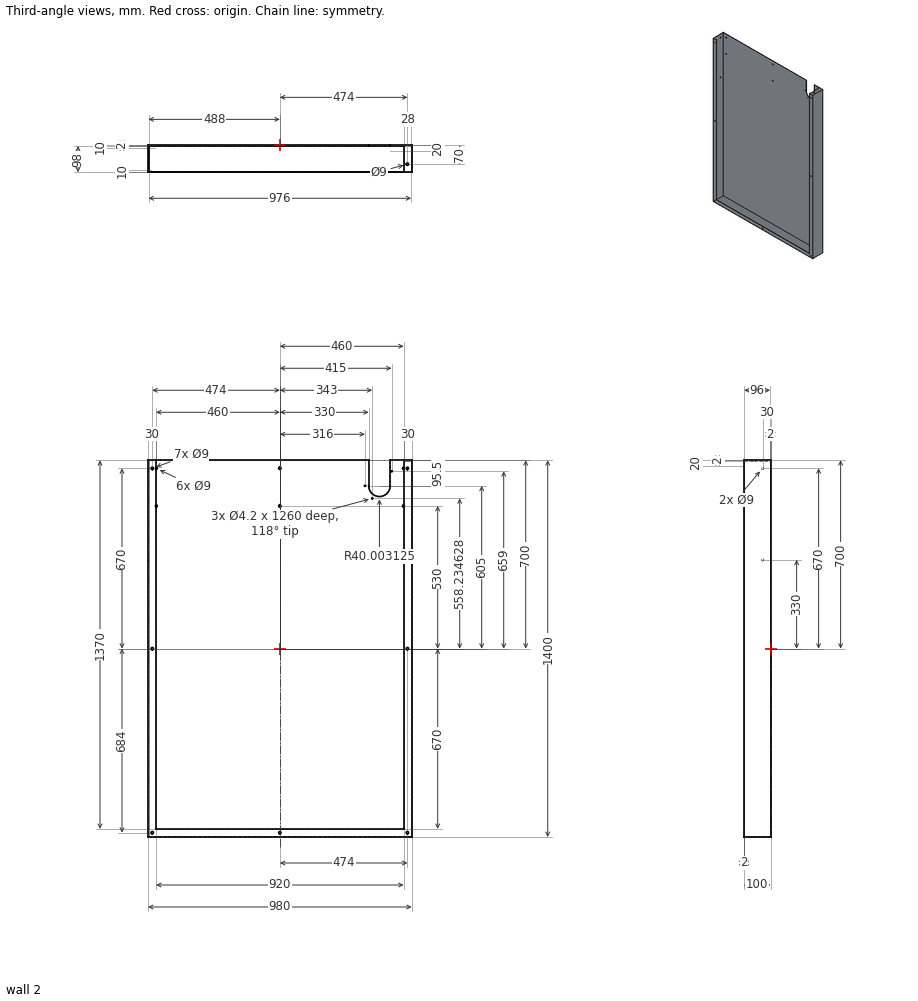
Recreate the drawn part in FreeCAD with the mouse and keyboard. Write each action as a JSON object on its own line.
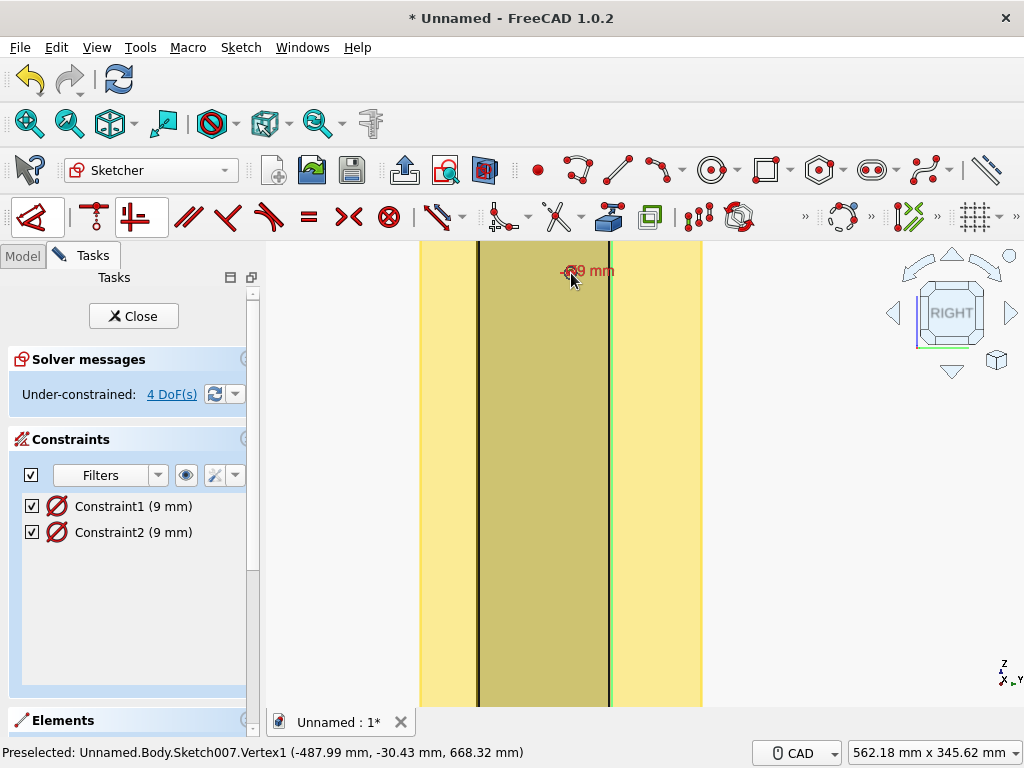
{"action": "key", "text": "l"}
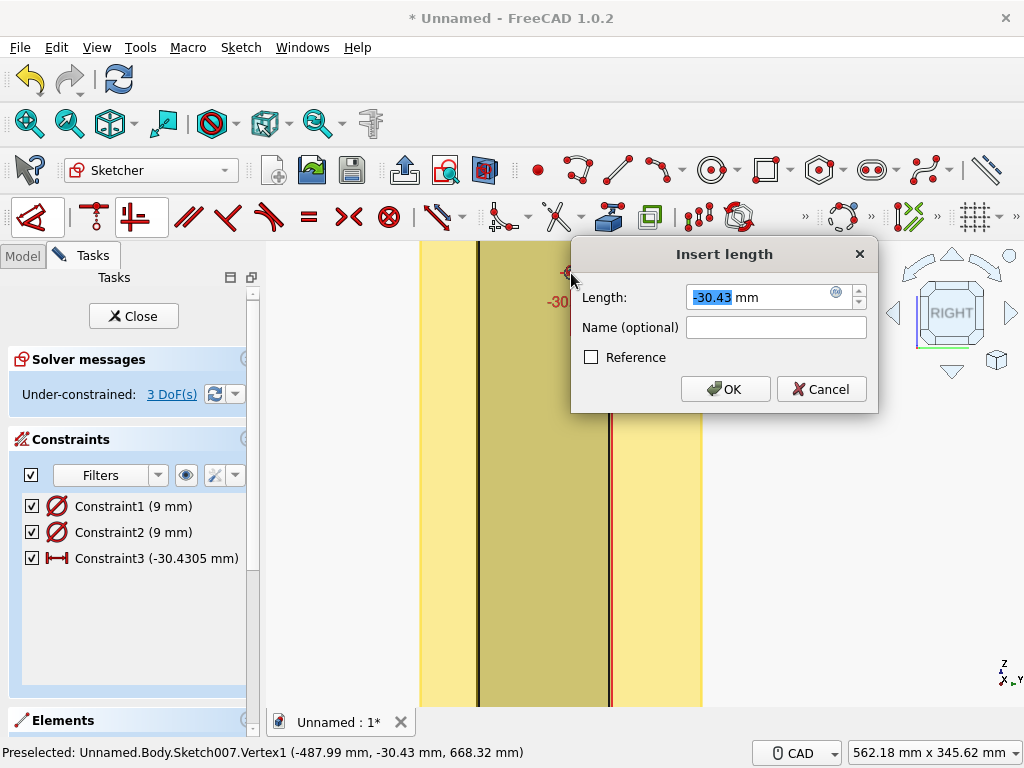
{"action": "type", "text": "-30"}
{"action": "key", "text": "Return"}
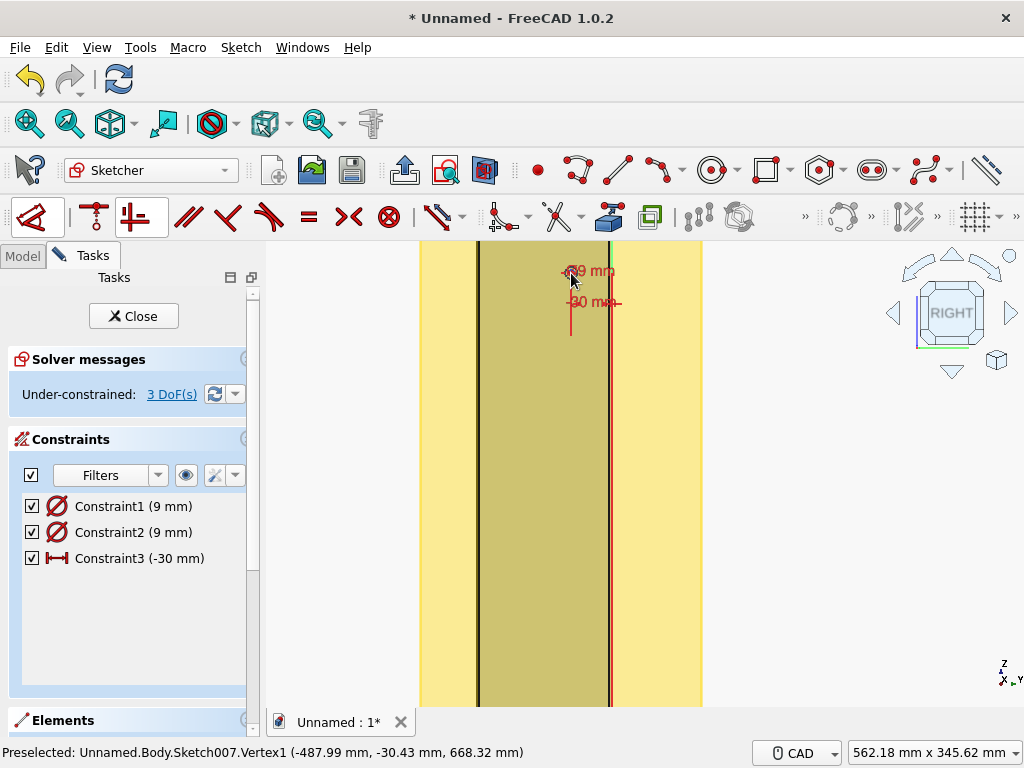
{"action": "scroll", "coordinate": [571, 368], "scroll_direction": "down", "scroll_amount": 6}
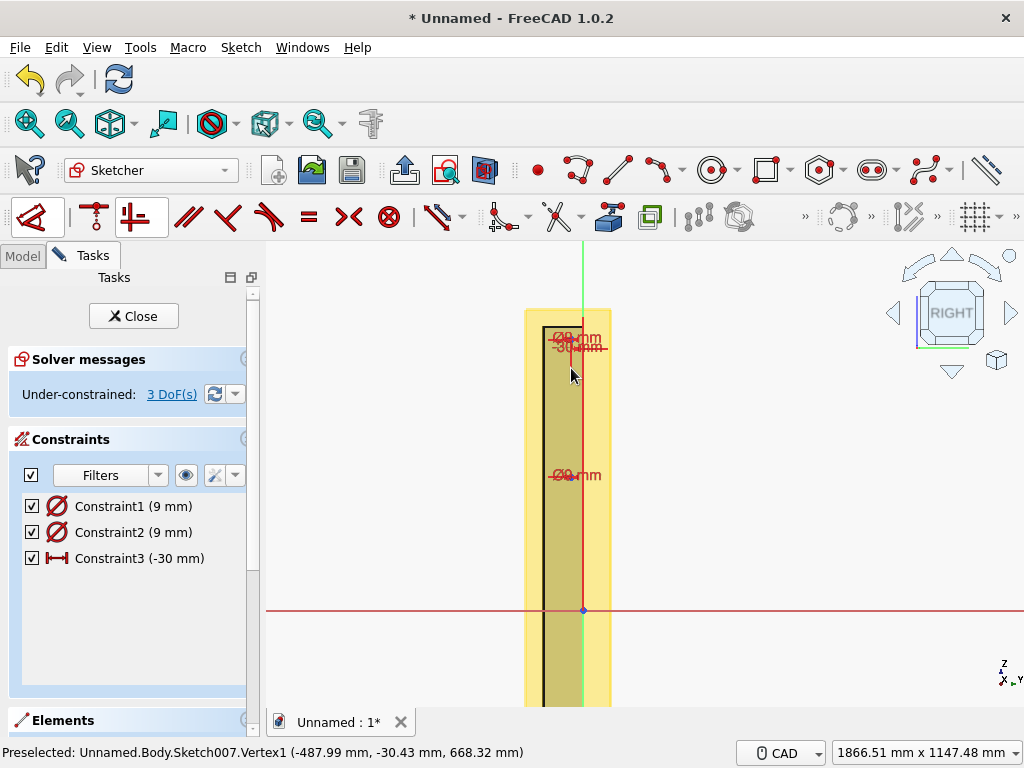
{"action": "scroll", "coordinate": [571, 477], "scroll_direction": "up", "scroll_amount": 6}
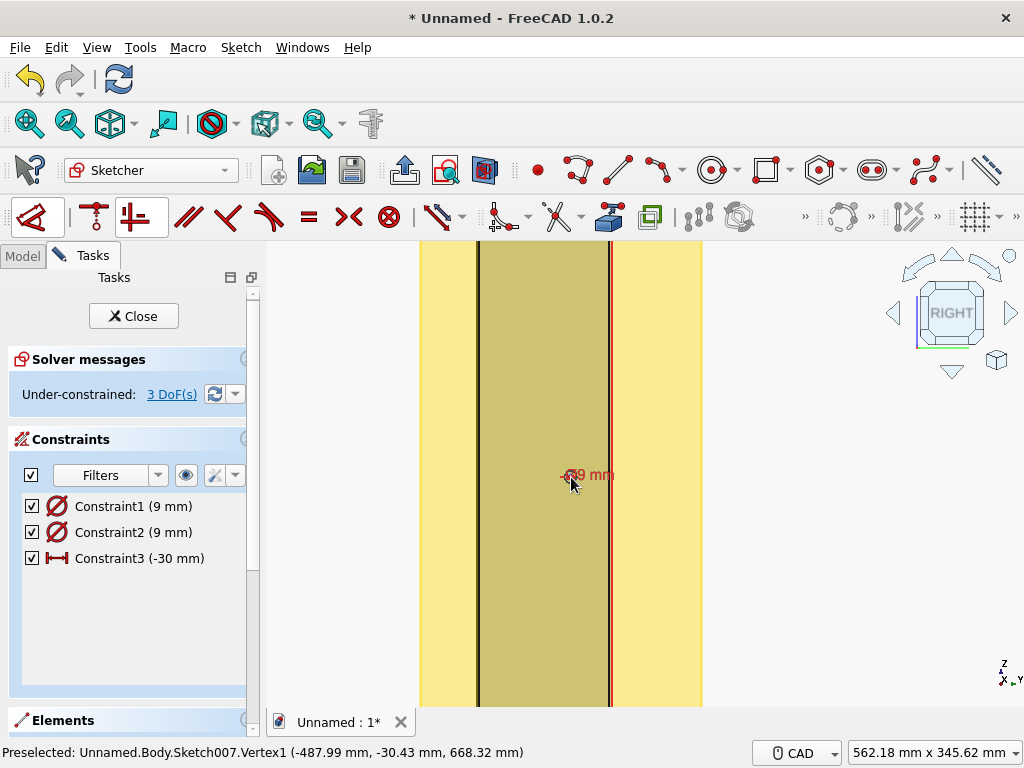
{"action": "left_click", "coordinate": [571, 477]}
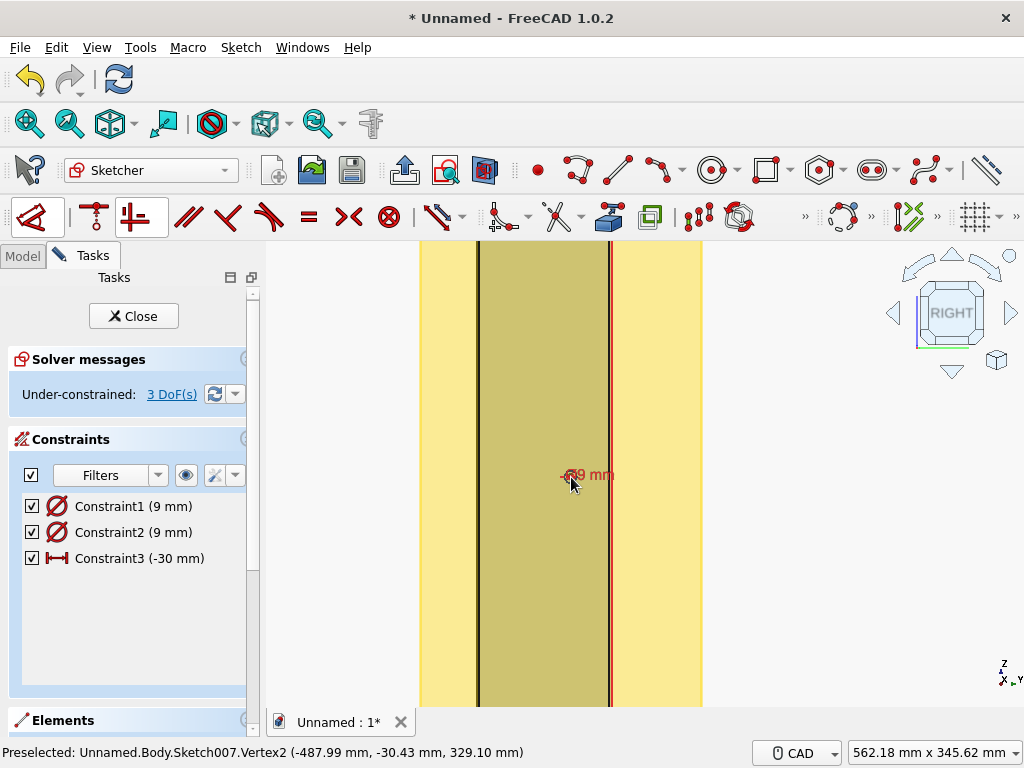
{"action": "left_click", "coordinate": [58, 218]}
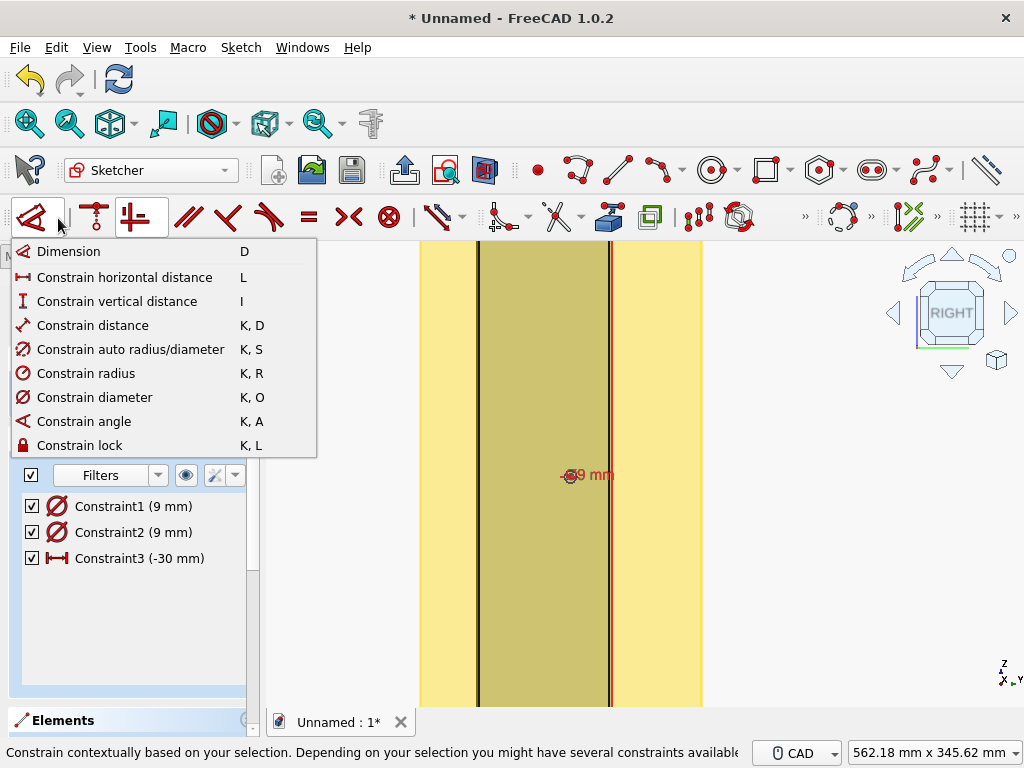
{"action": "left_click", "coordinate": [164, 277]}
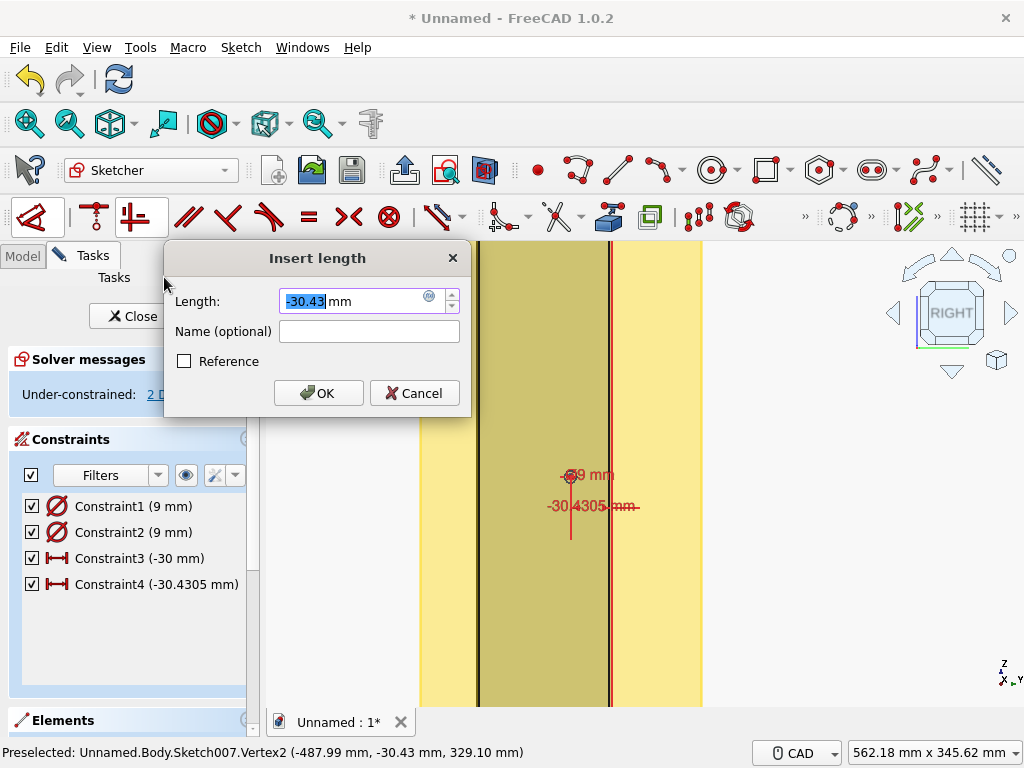
{"action": "type", "text": "-30"}
{"action": "key", "text": "Return"}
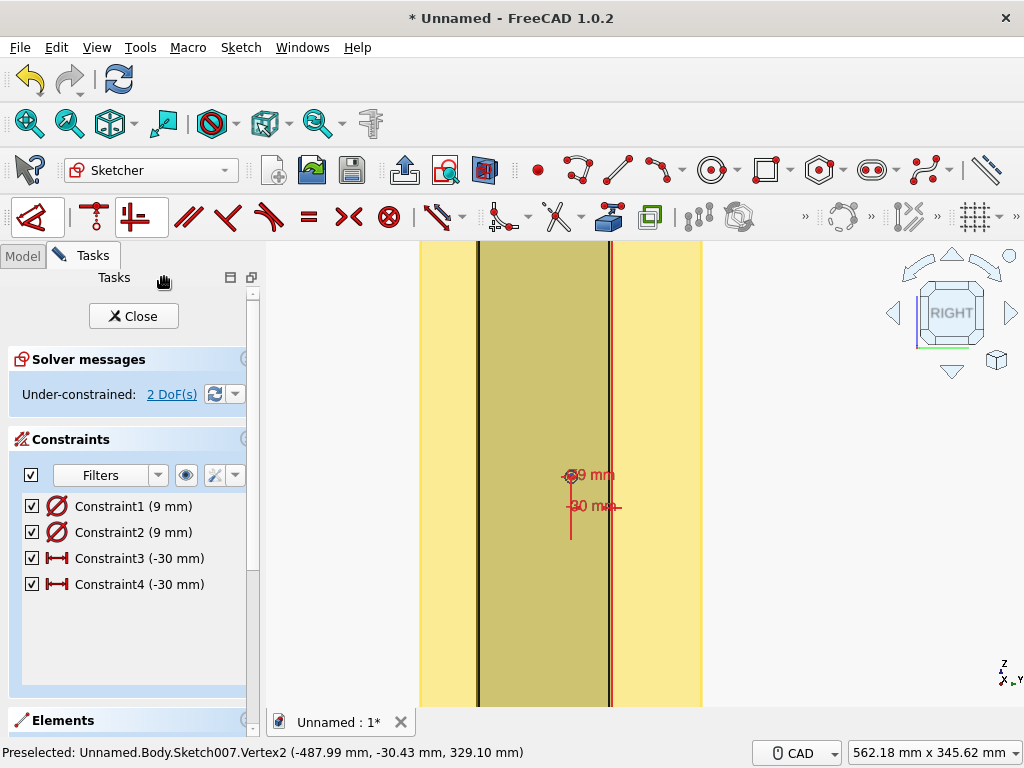
{"action": "scroll", "coordinate": [571, 477], "scroll_direction": "down", "scroll_amount": 6}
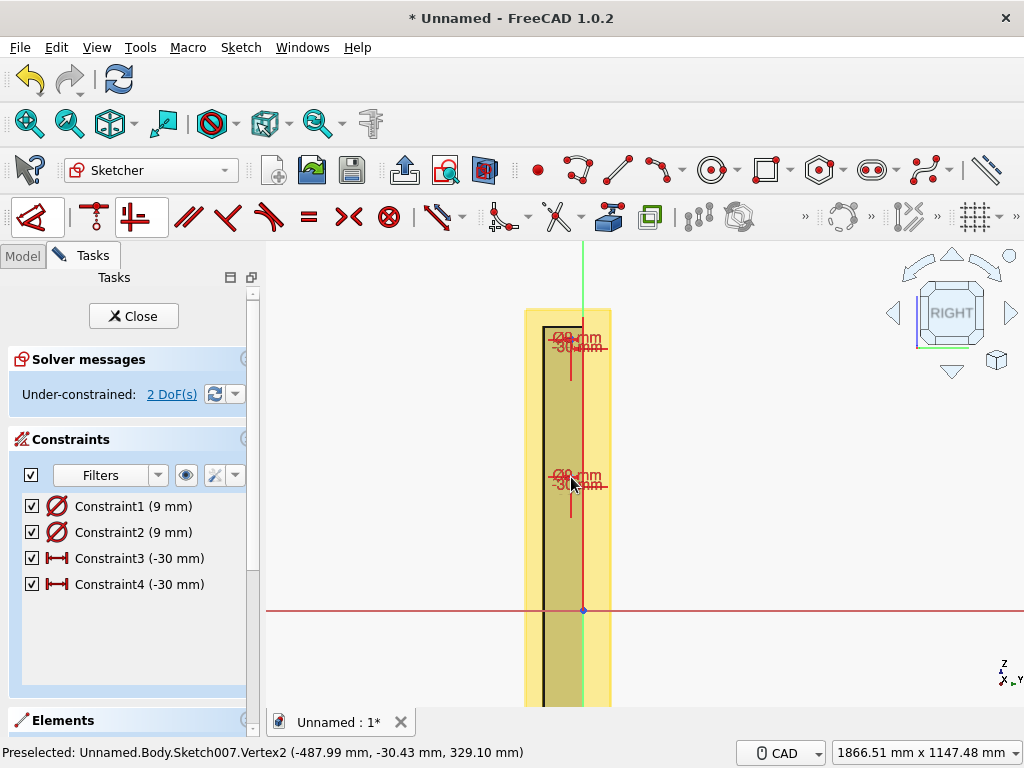
{"action": "left_click", "coordinate": [571, 340]}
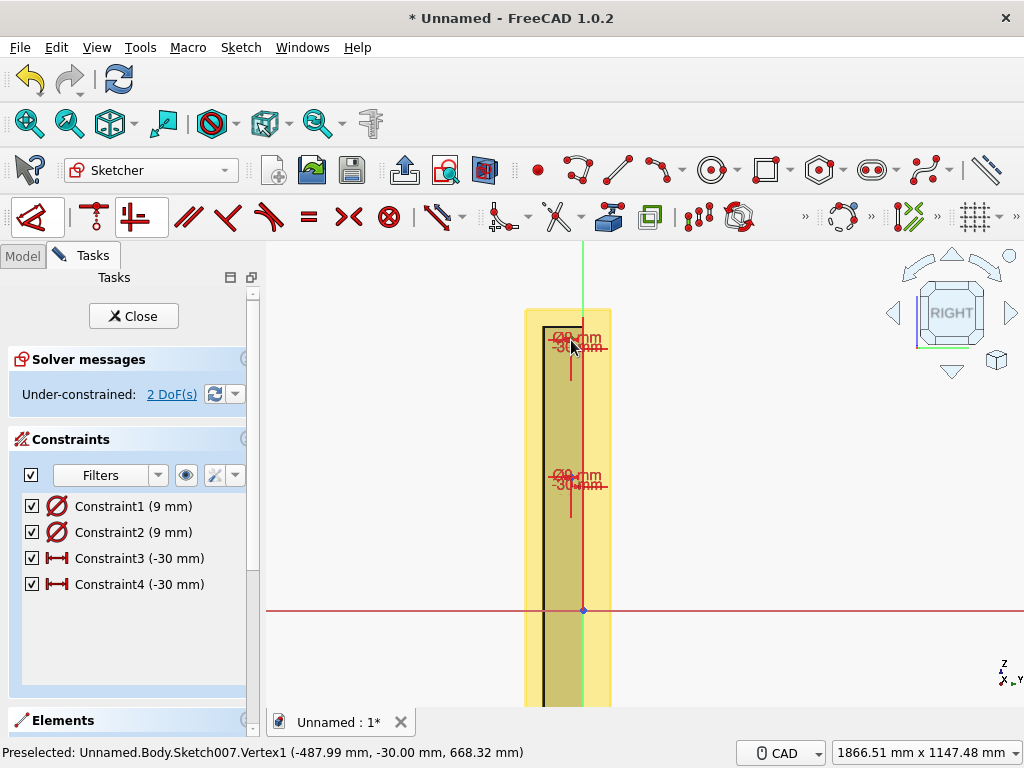
{"action": "key", "text": "i"}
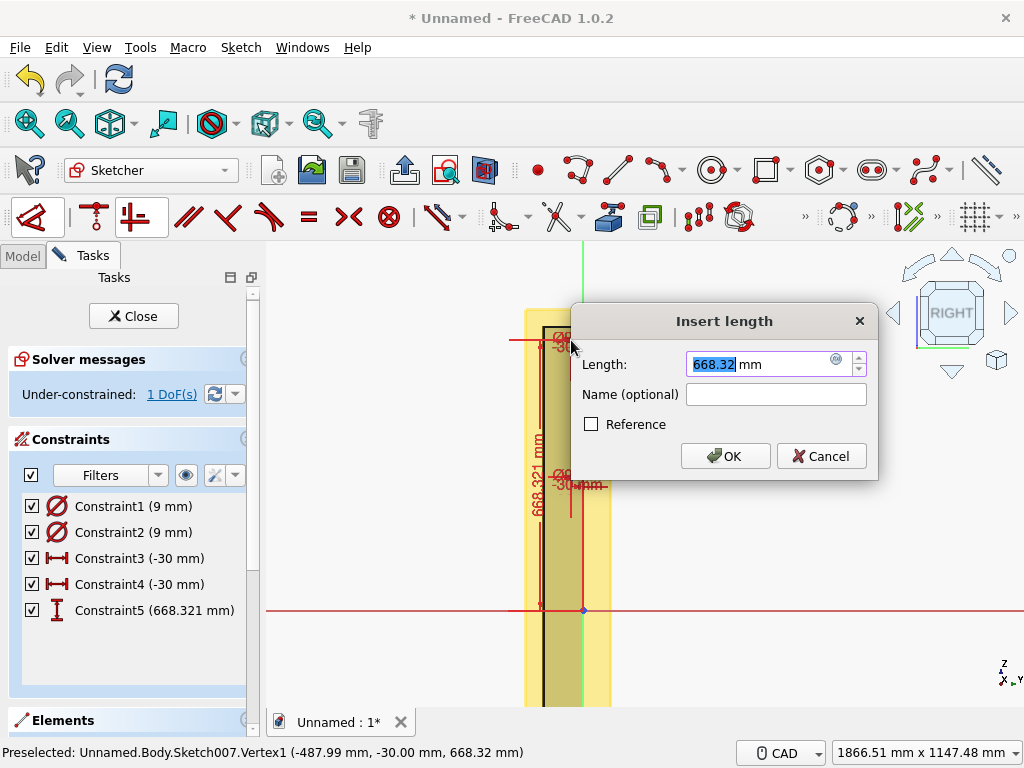
{"action": "type", "text": "670"}
{"action": "key", "text": "Return"}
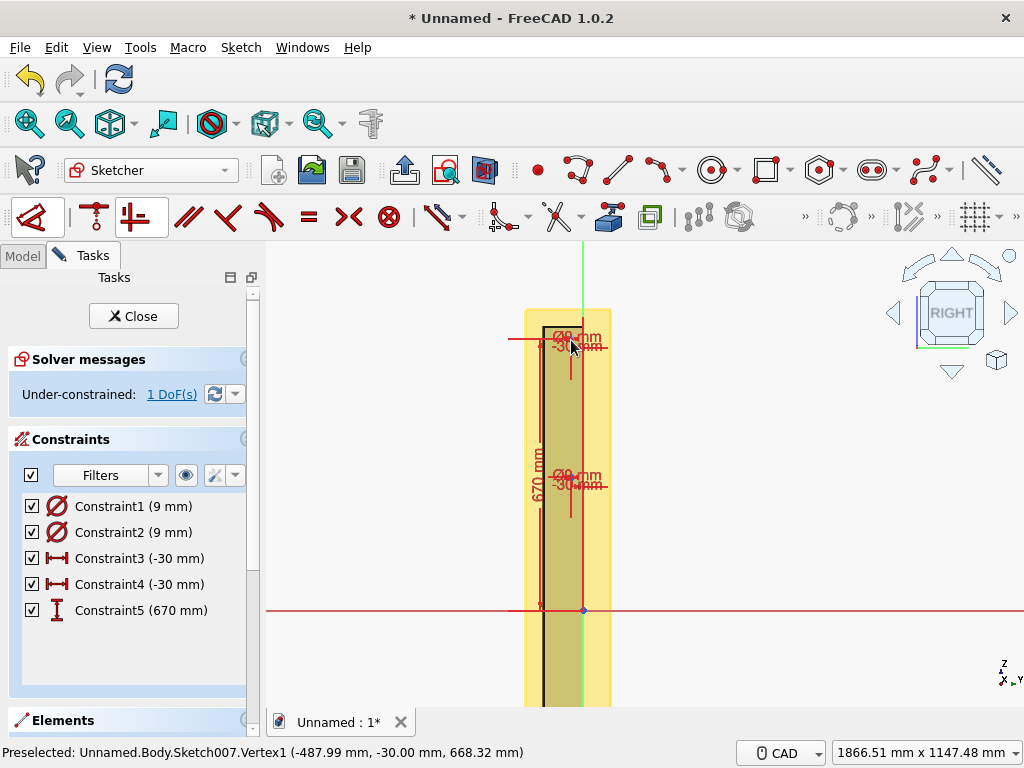
{"action": "left_click", "coordinate": [571, 477]}